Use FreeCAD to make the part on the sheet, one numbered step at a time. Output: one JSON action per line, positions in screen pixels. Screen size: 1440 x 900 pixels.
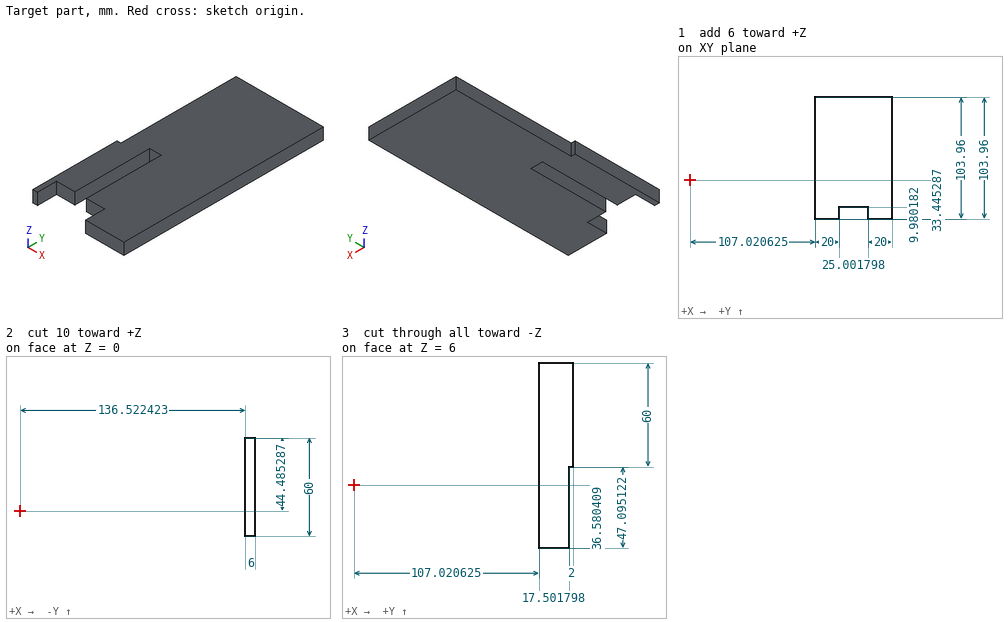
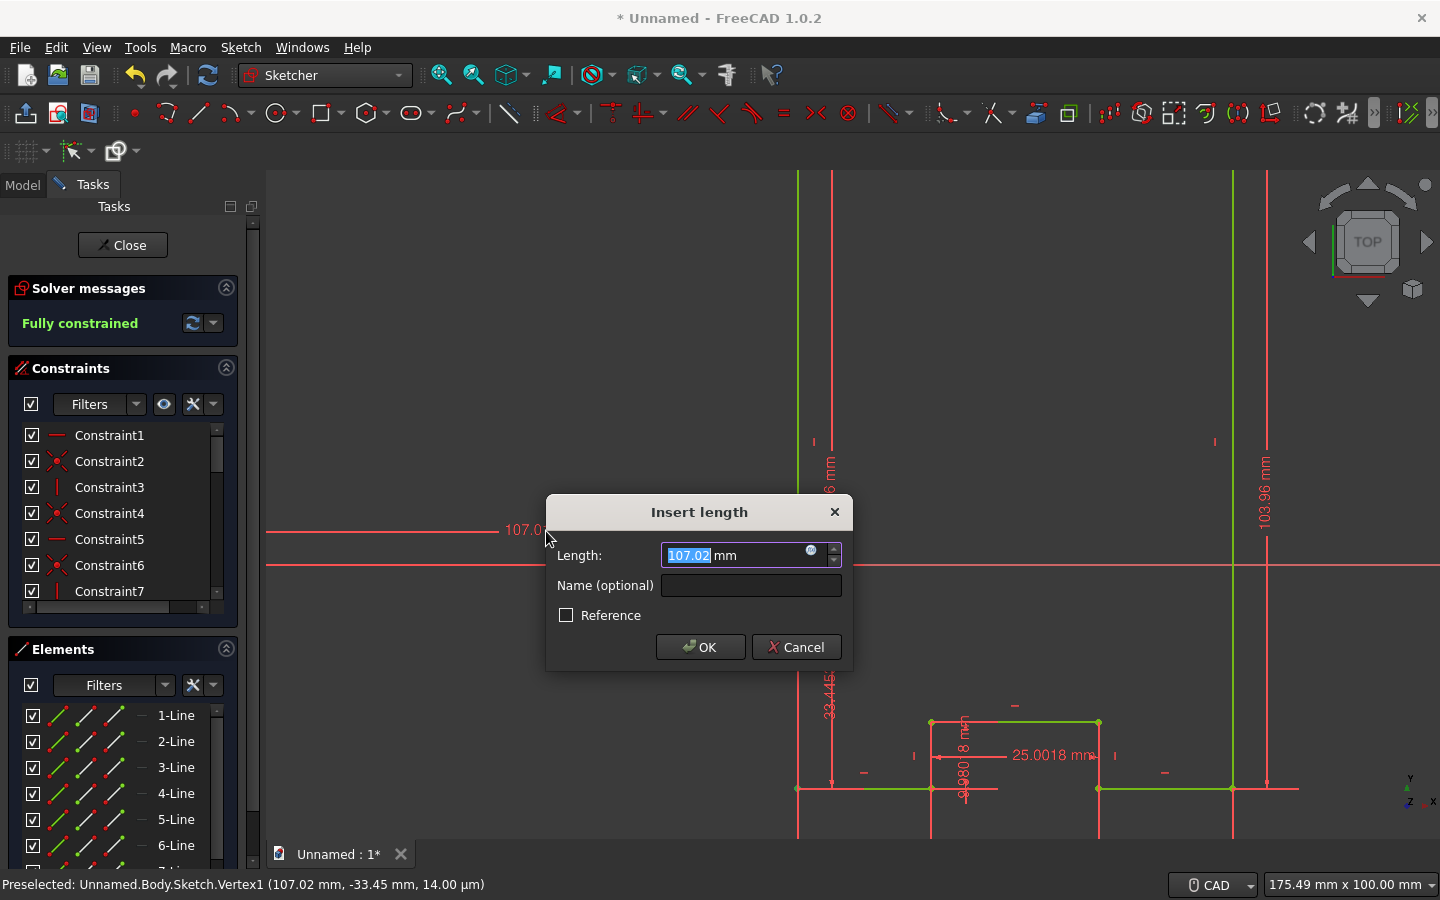
{"action": "type", "text": "107.020625"}
{"action": "key", "text": "Return"}
{"action": "key", "text": "Escape"}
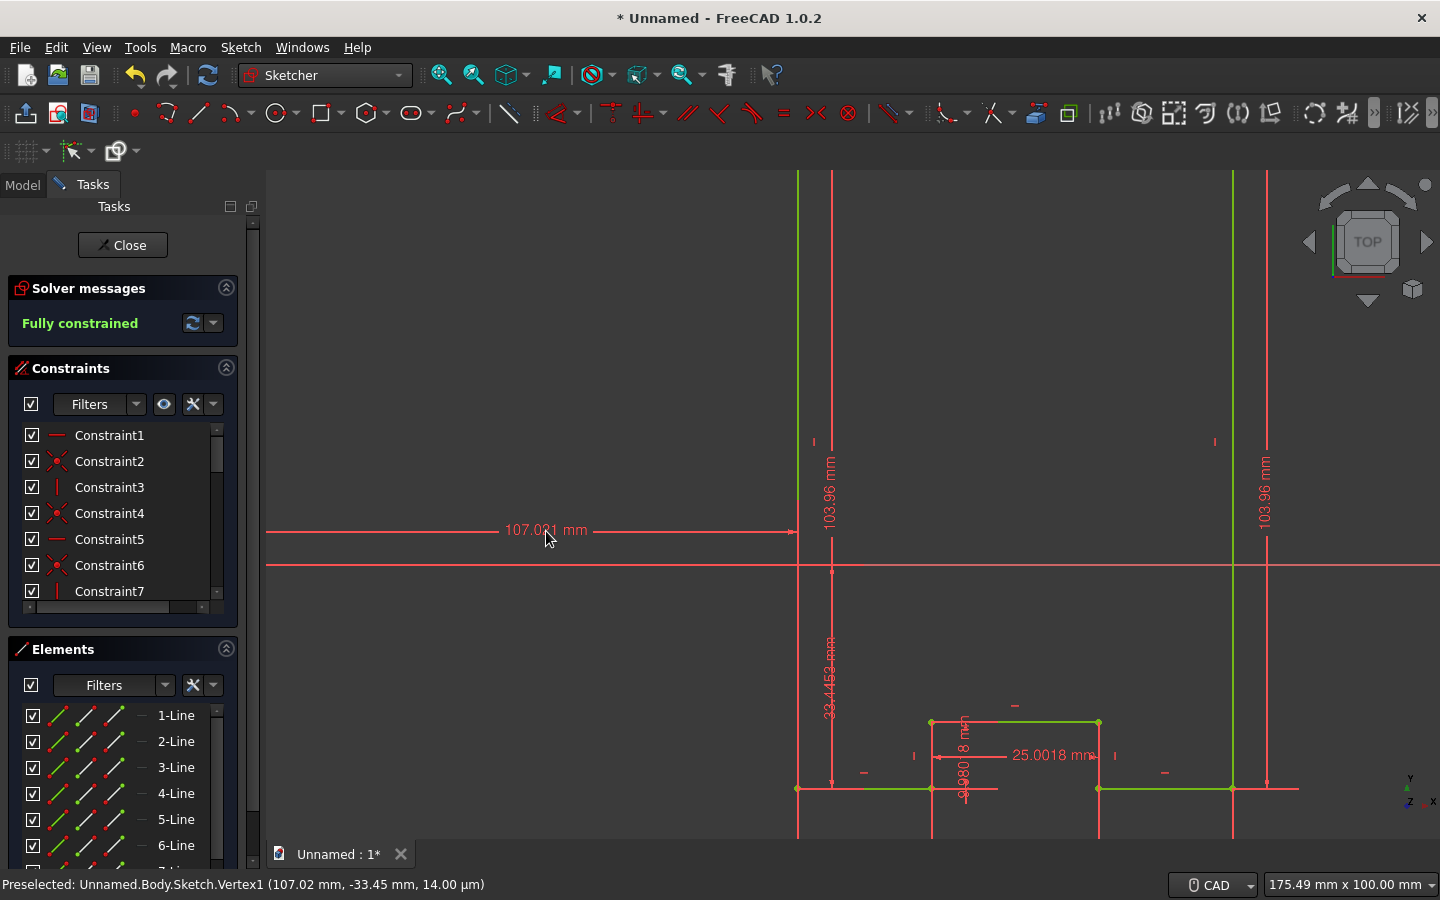
{"action": "left_click", "coordinate": [123, 245]}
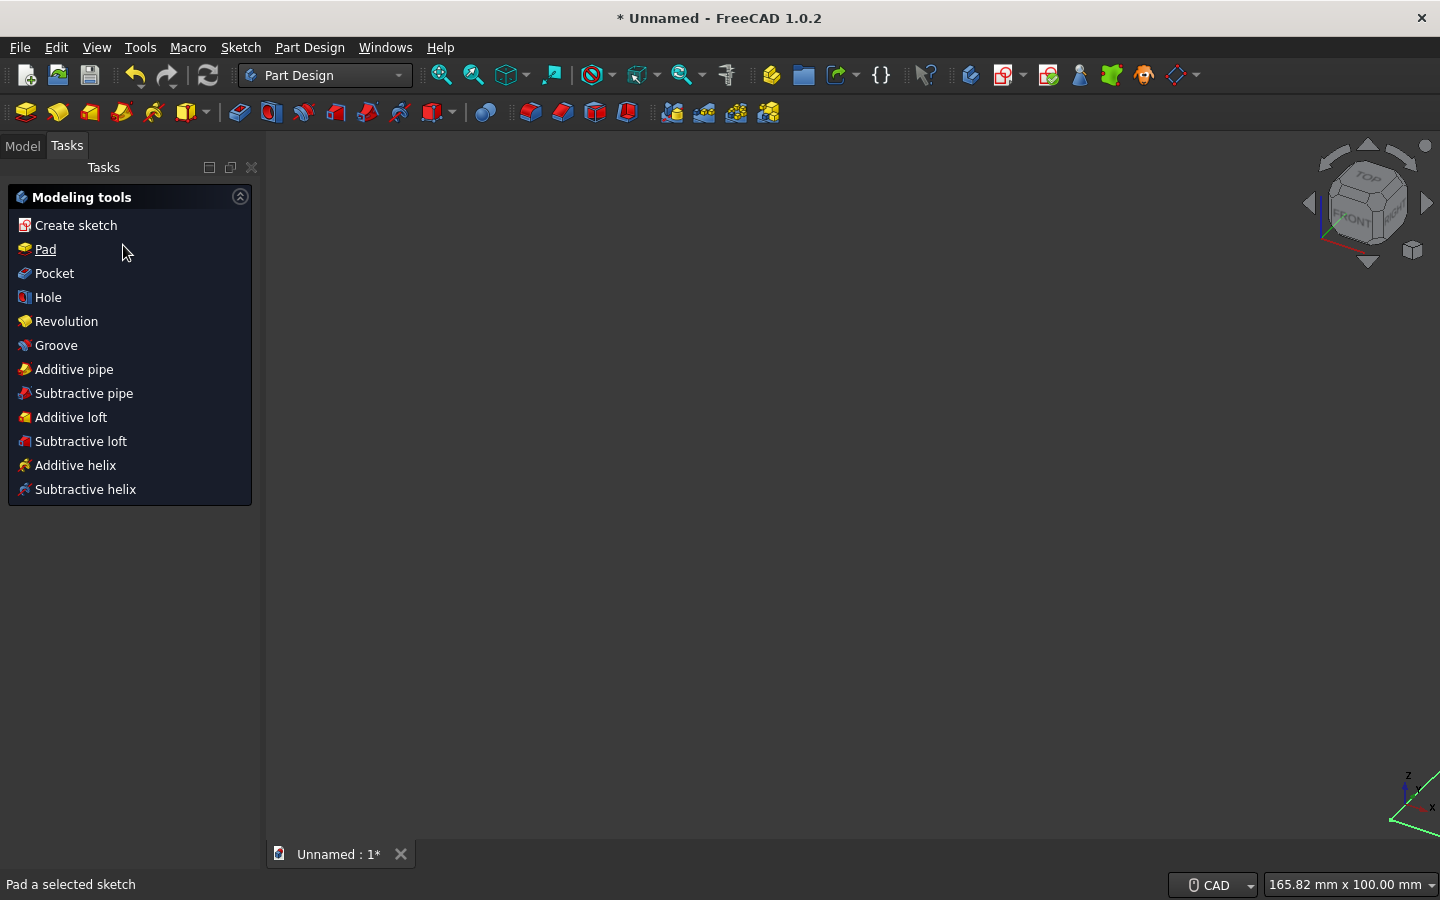
{"action": "left_click", "coordinate": [26, 112]}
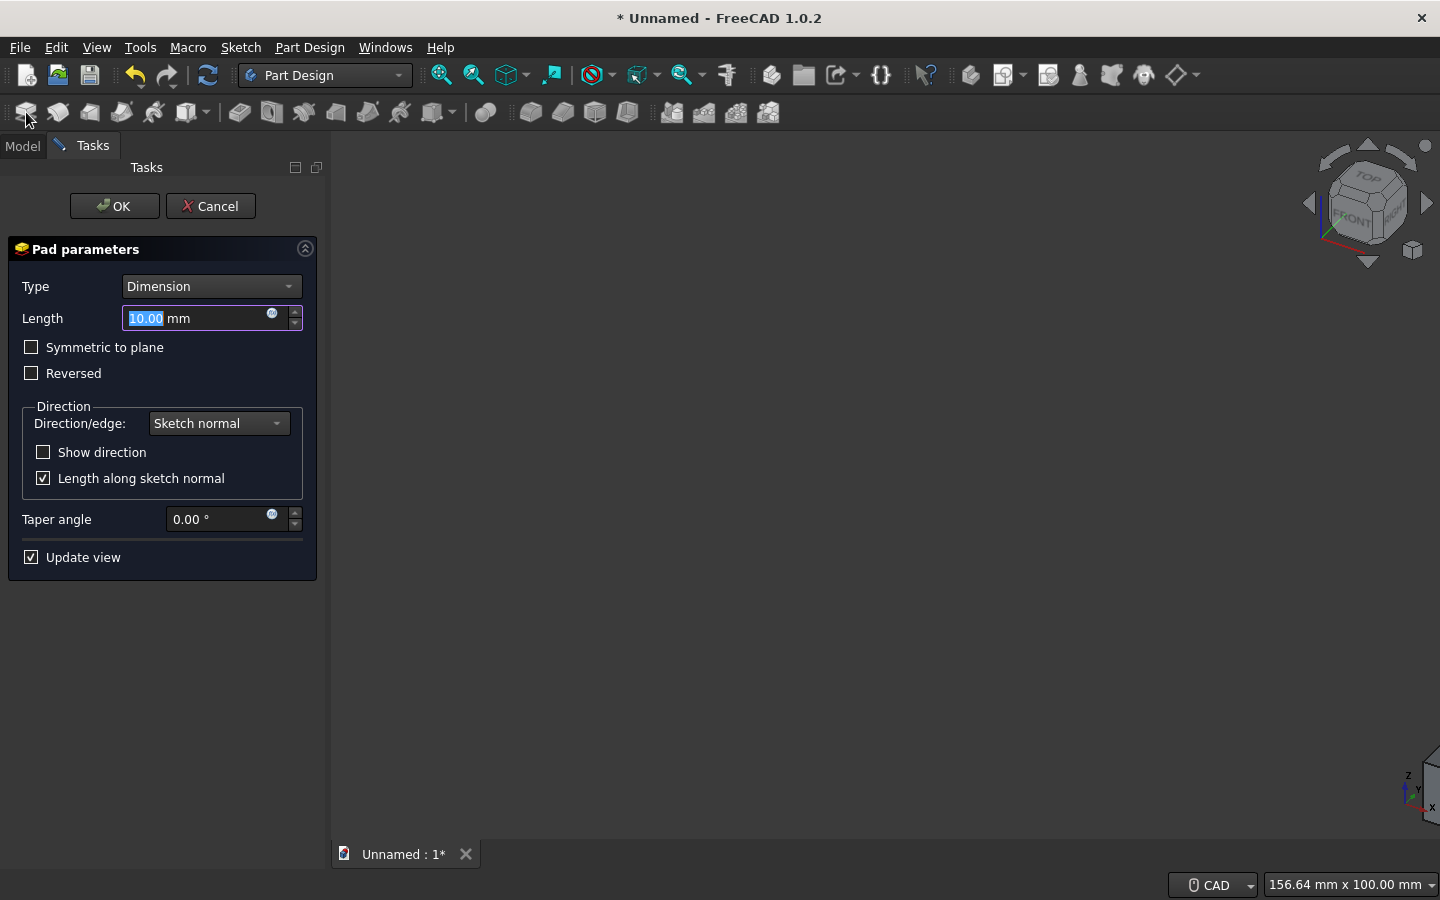
{"action": "type", "text": "6"}
{"action": "key", "text": "Tab"}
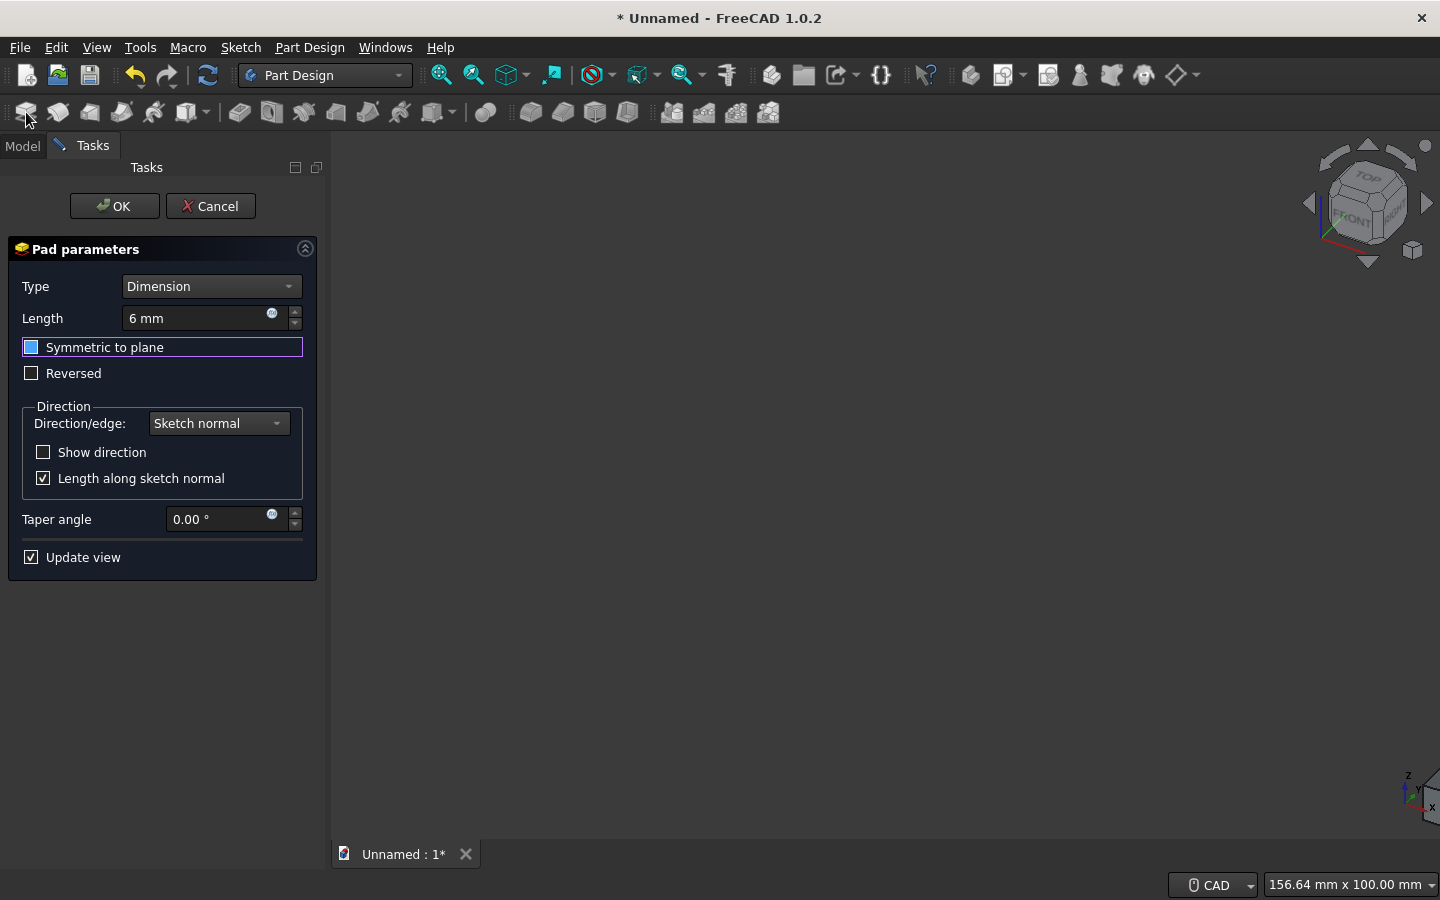
{"action": "left_click", "coordinate": [115, 206]}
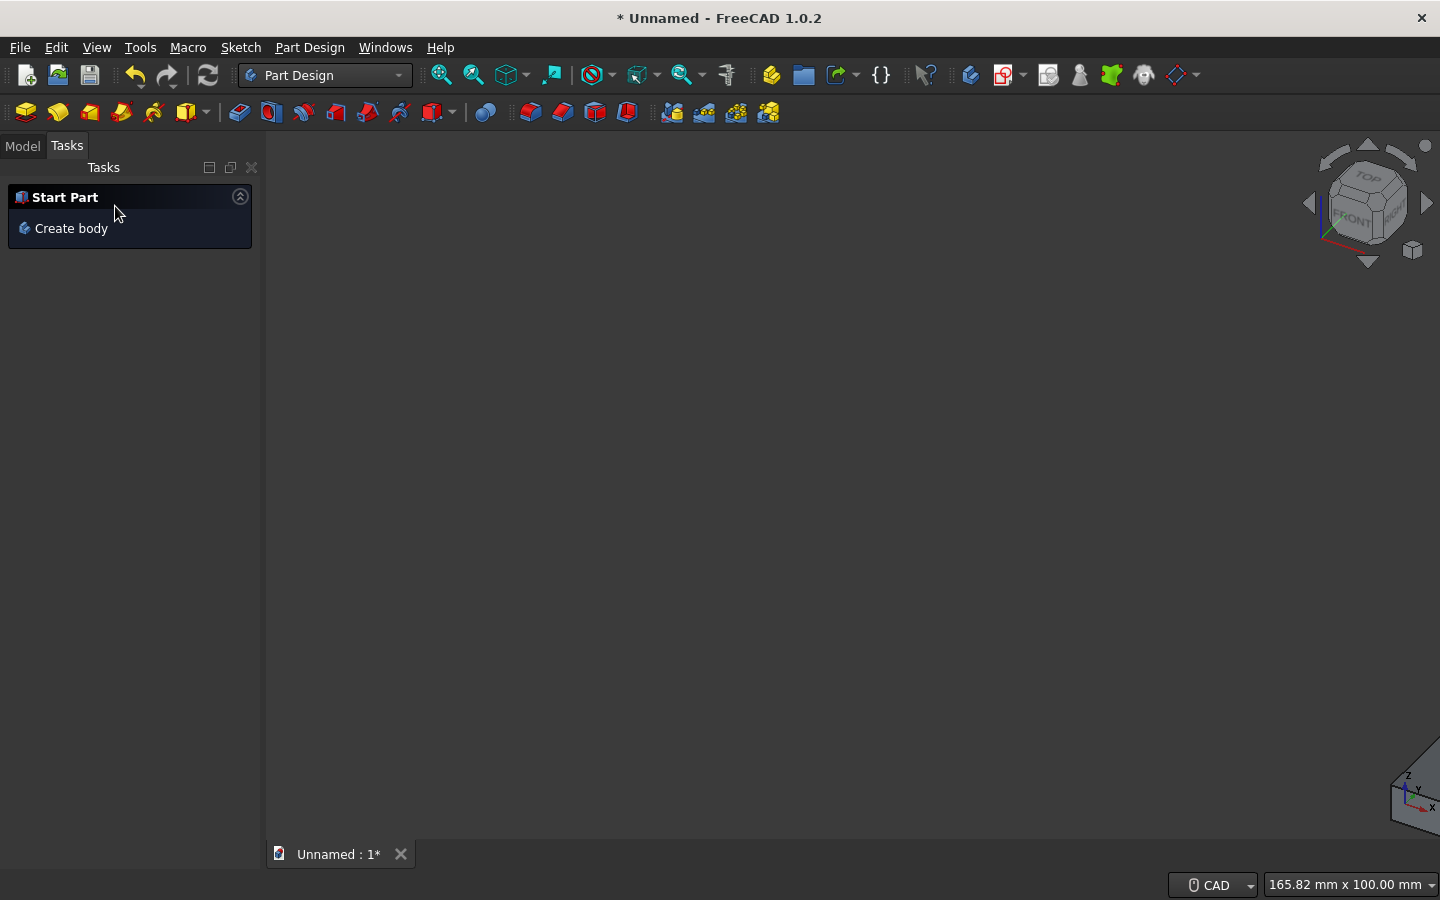
{"action": "left_click", "coordinate": [442, 76]}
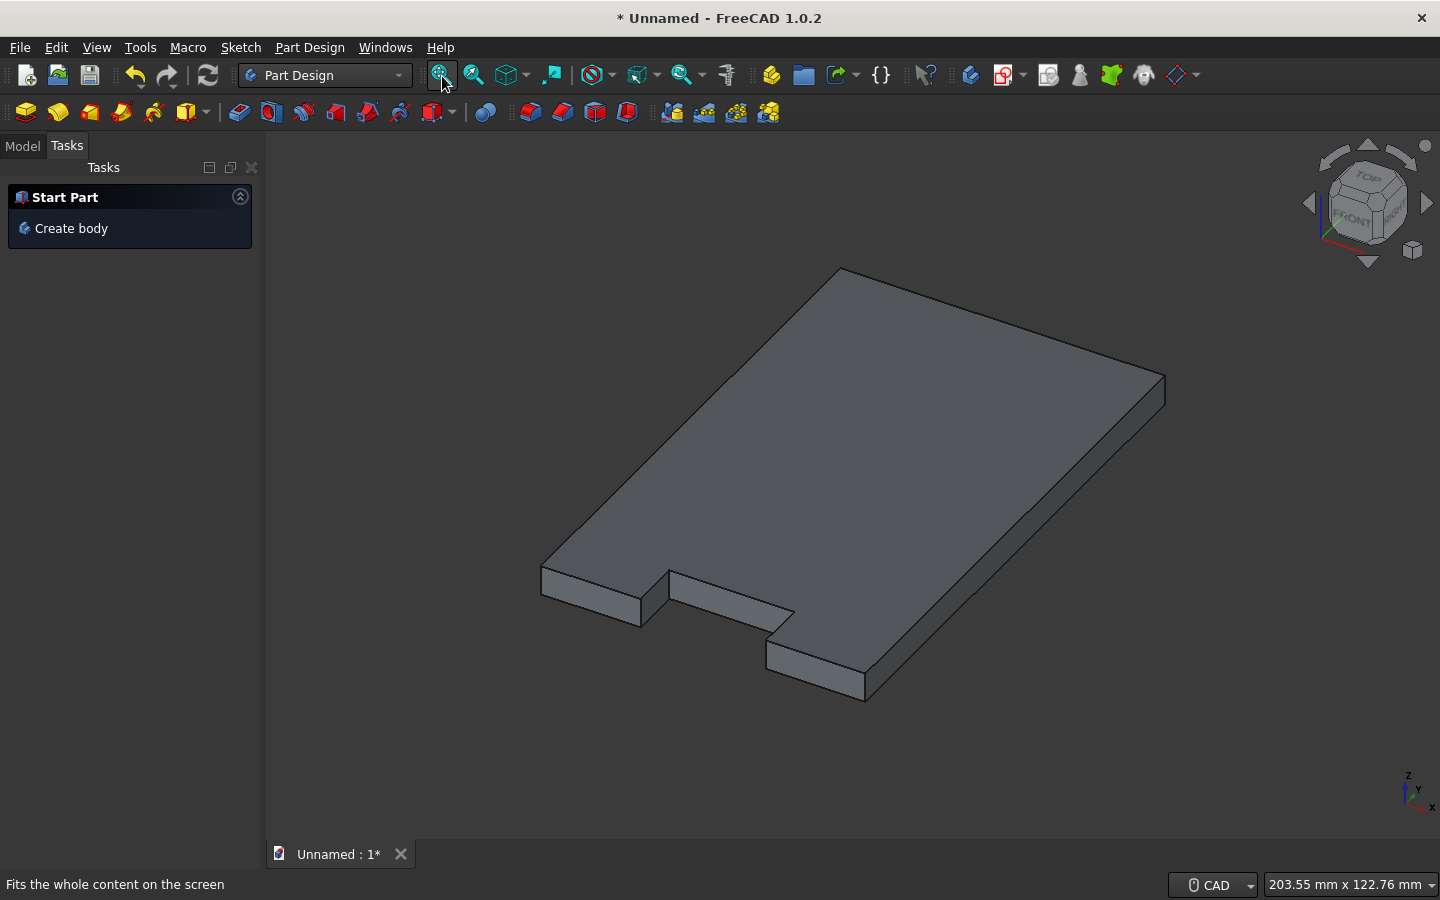
{"action": "key", "text": "5"}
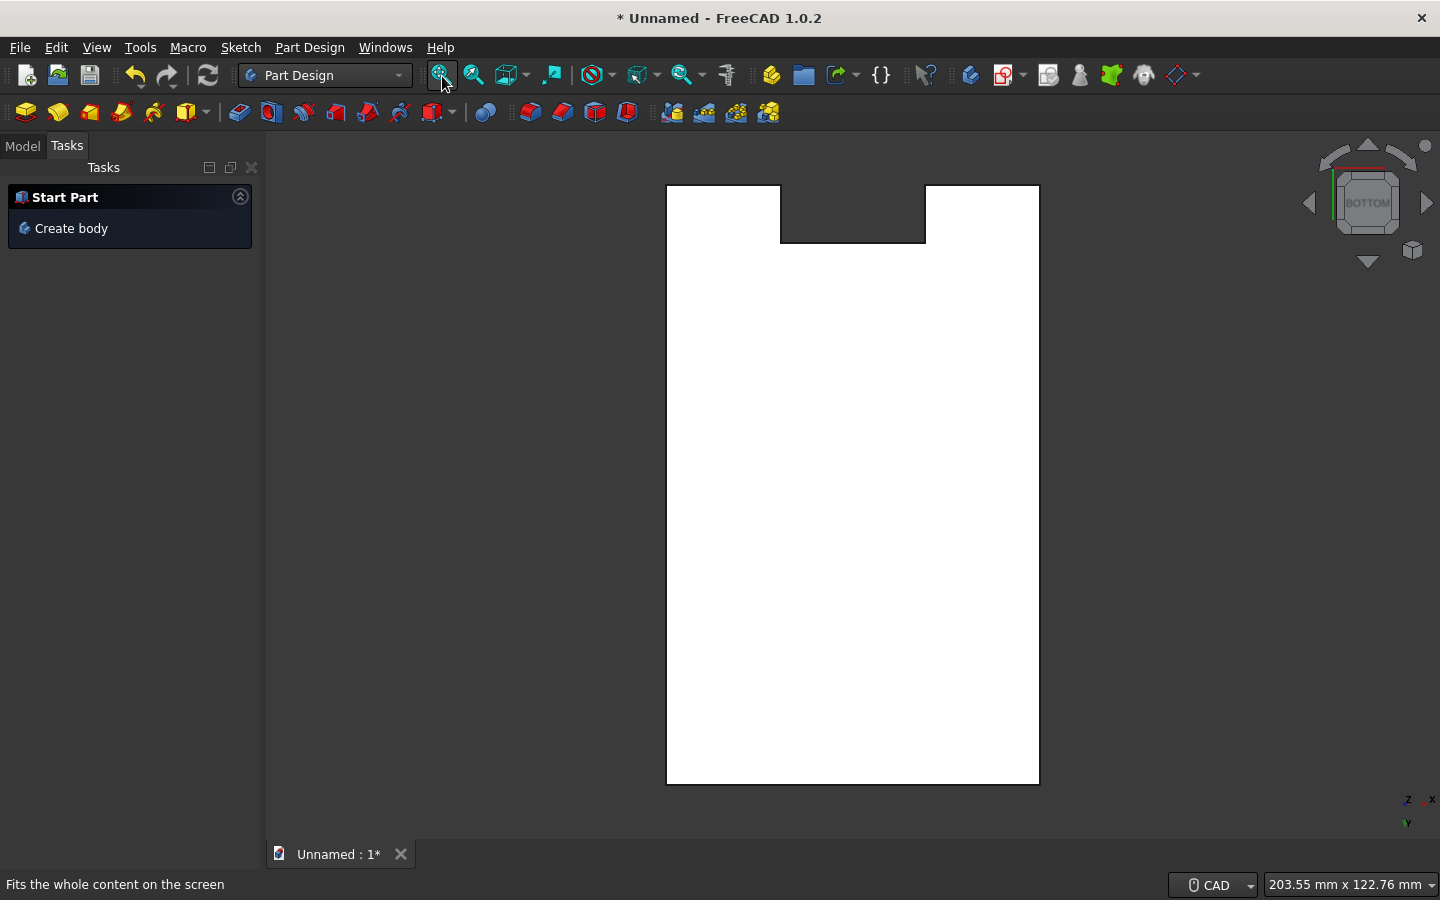
{"action": "left_click", "coordinate": [853, 570]}